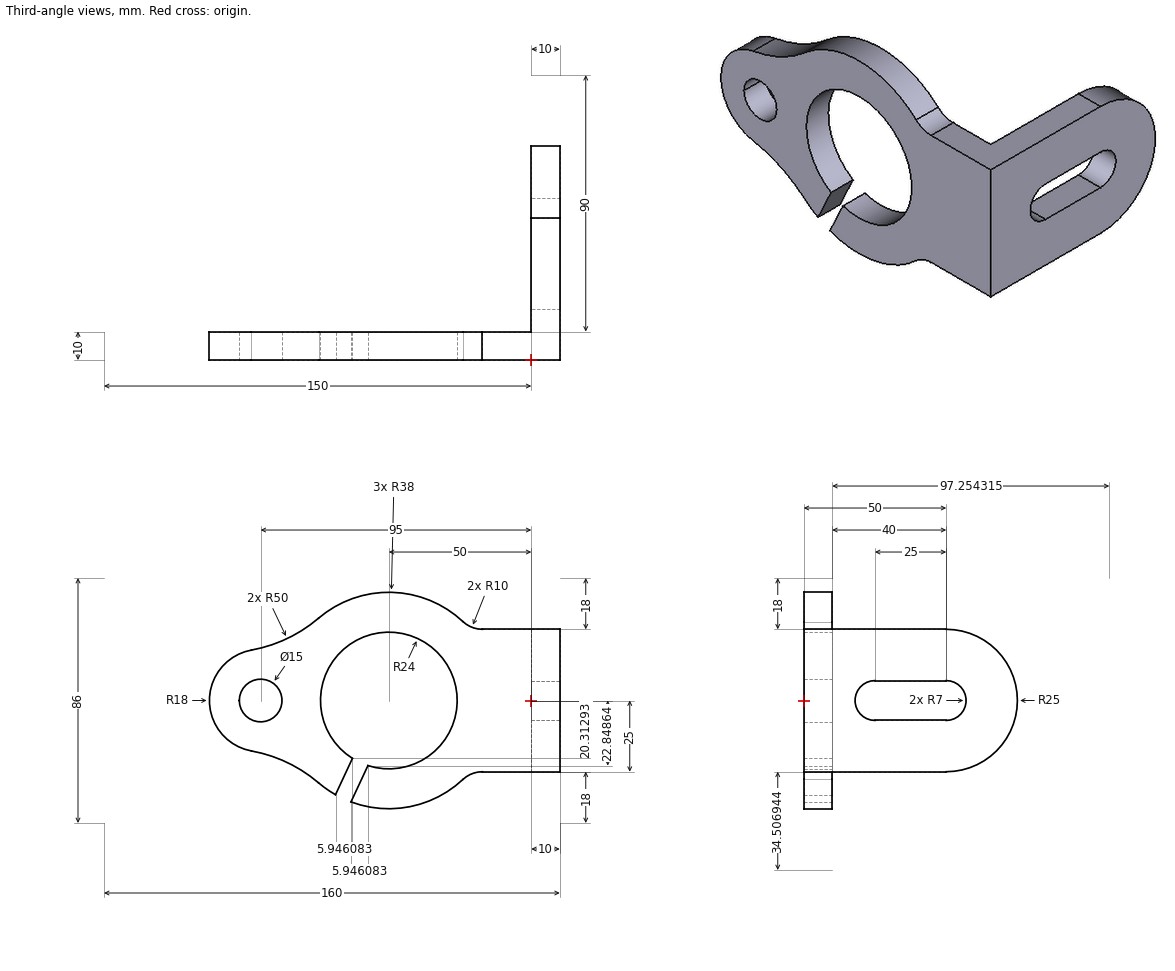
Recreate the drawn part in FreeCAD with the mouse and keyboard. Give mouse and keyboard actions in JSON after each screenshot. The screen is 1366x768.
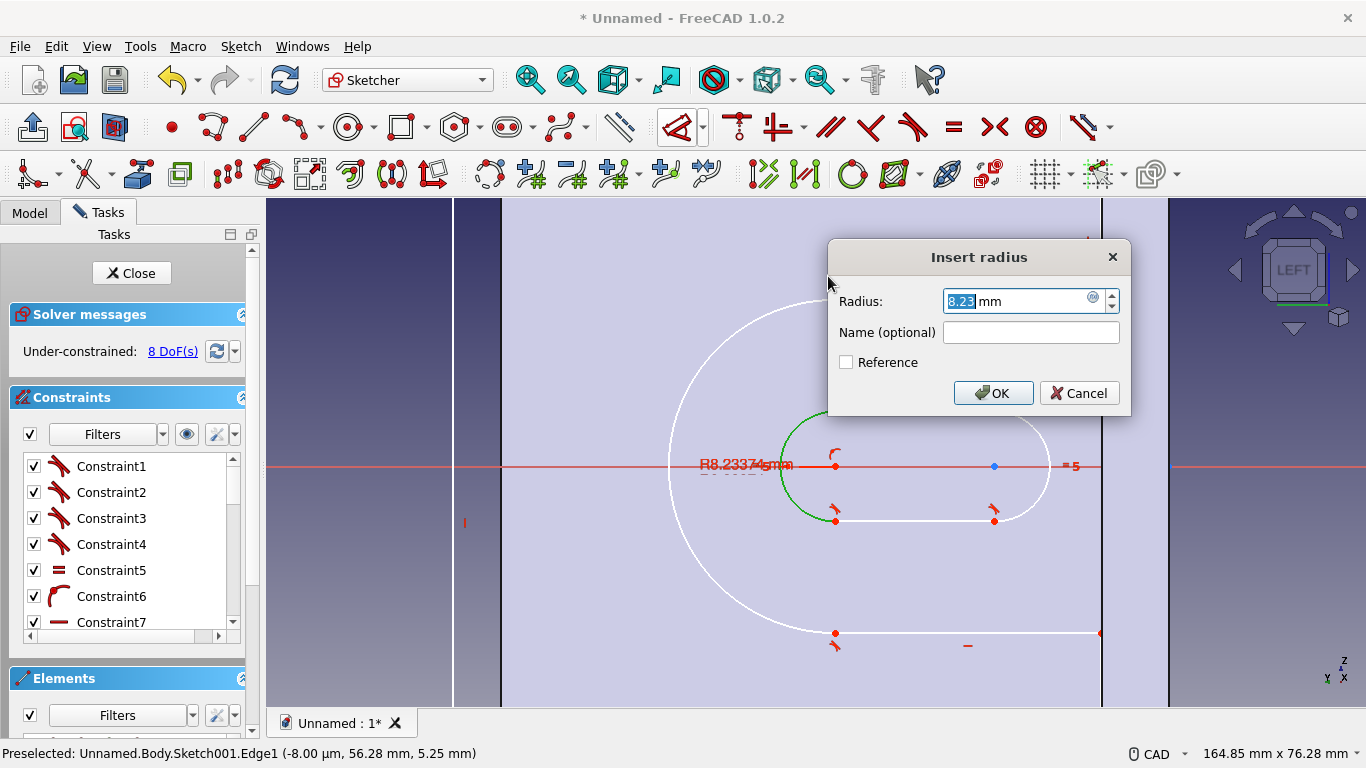
{"action": "type", "text": "7"}
{"action": "key", "text": "Return"}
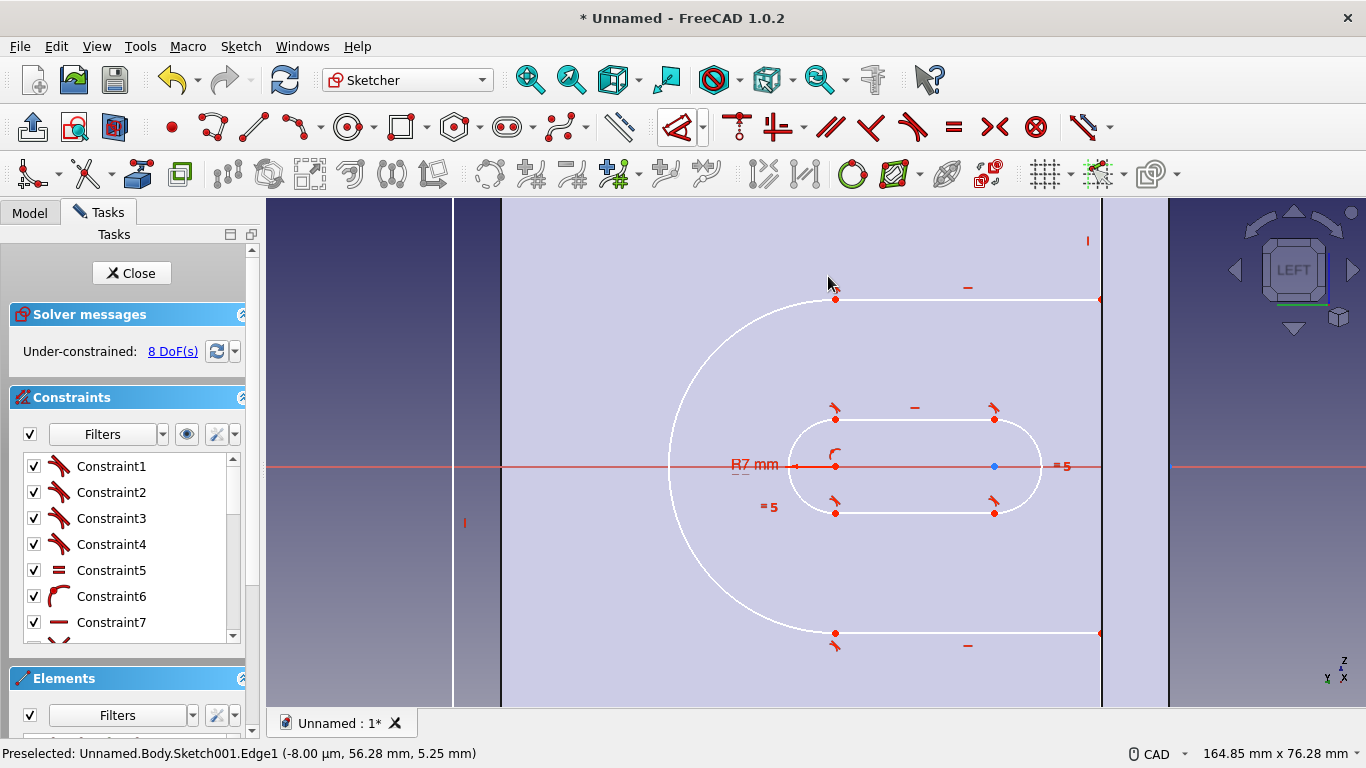
{"action": "left_click", "coordinate": [701, 369]}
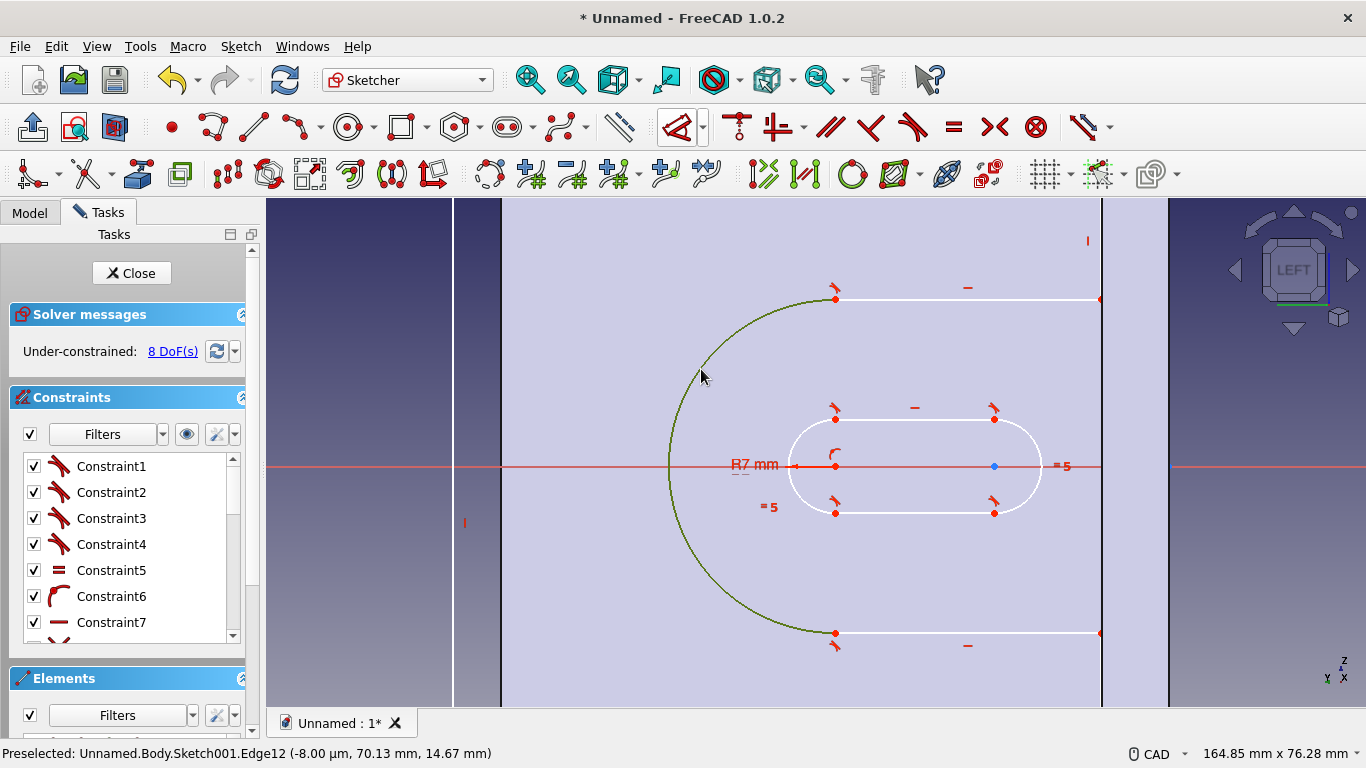
{"action": "left_click", "coordinate": [702, 128]}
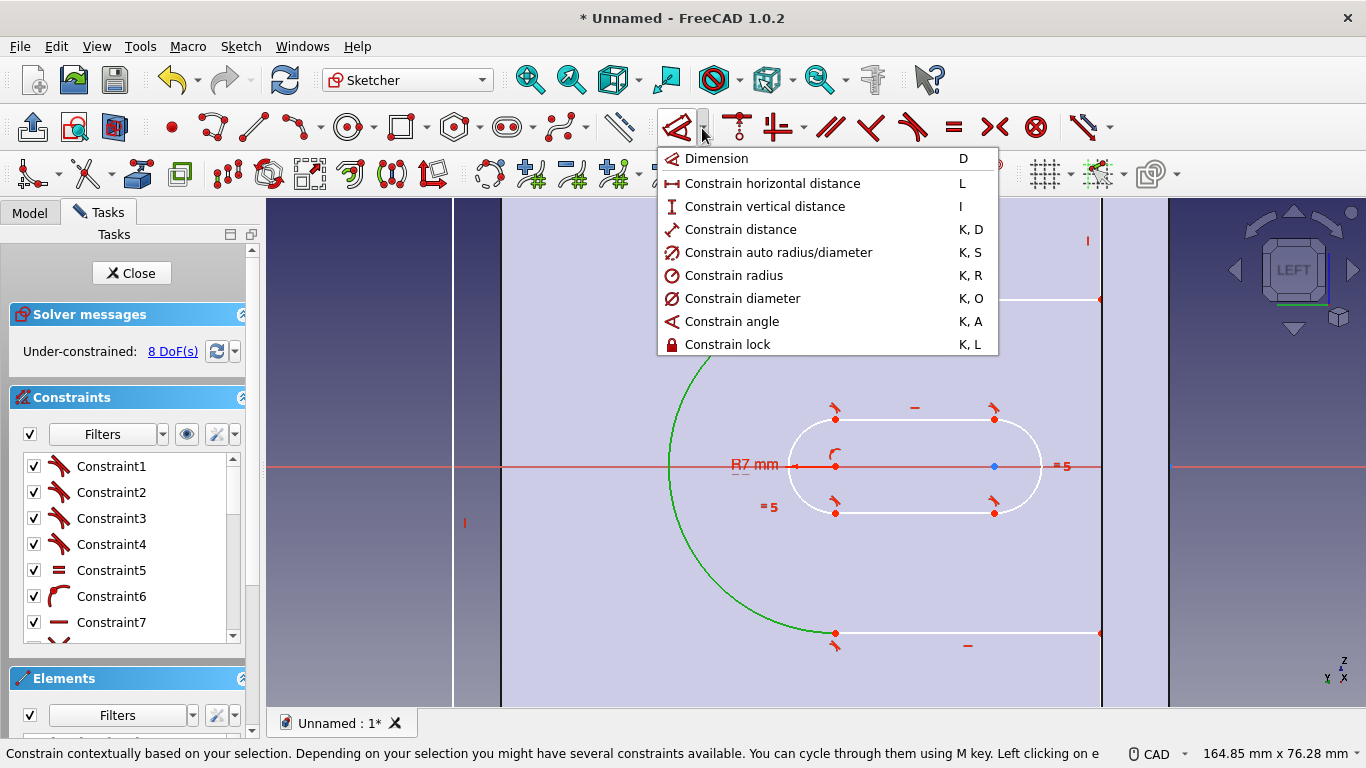
{"action": "left_click", "coordinate": [828, 276]}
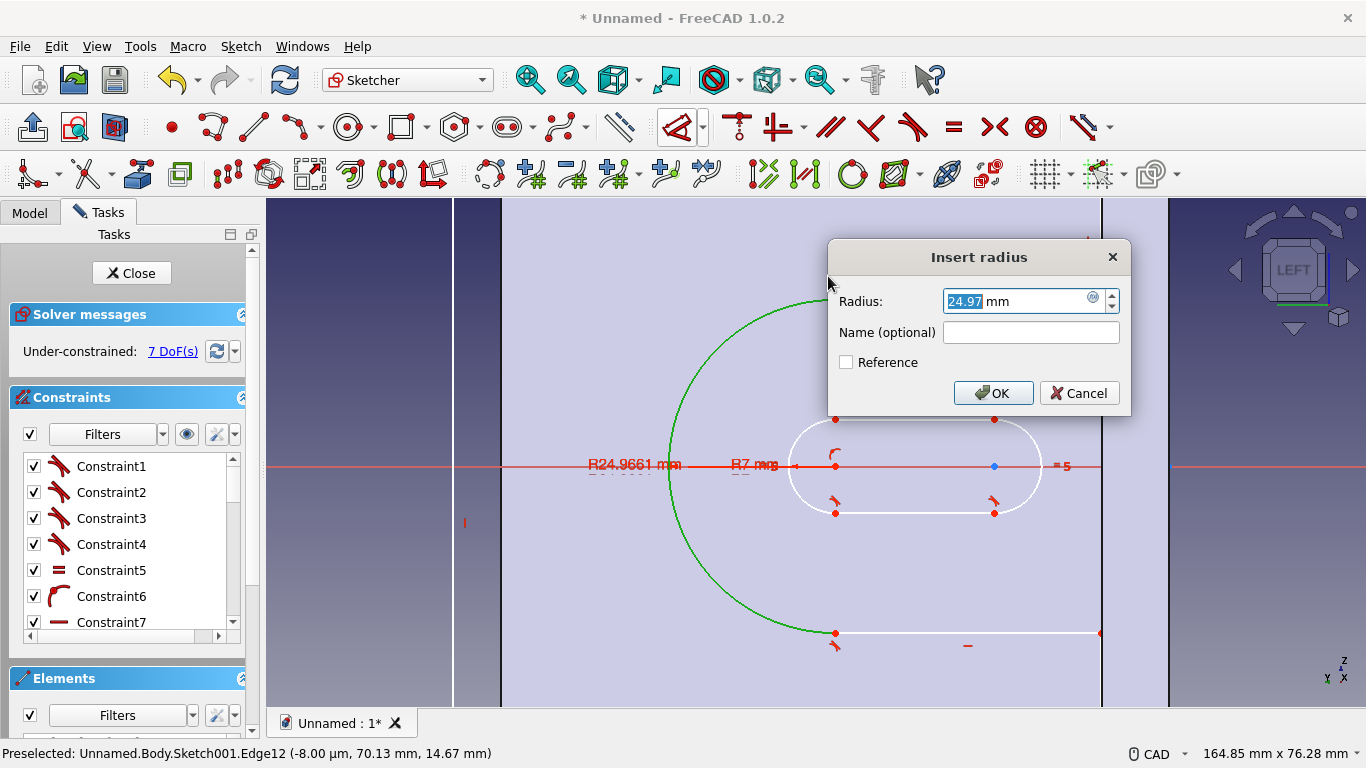
{"action": "type", "text": "25"}
{"action": "key", "text": "Return"}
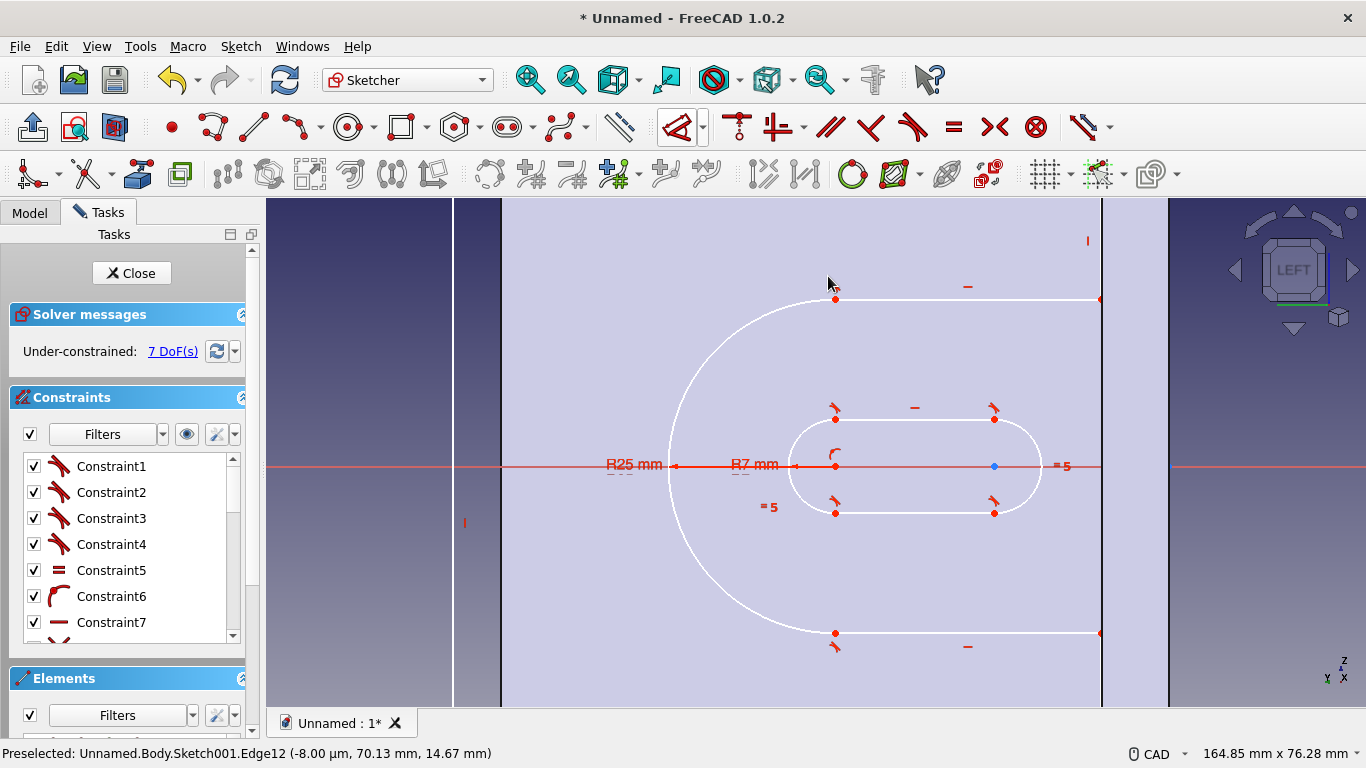
{"action": "left_click", "coordinate": [883, 420]}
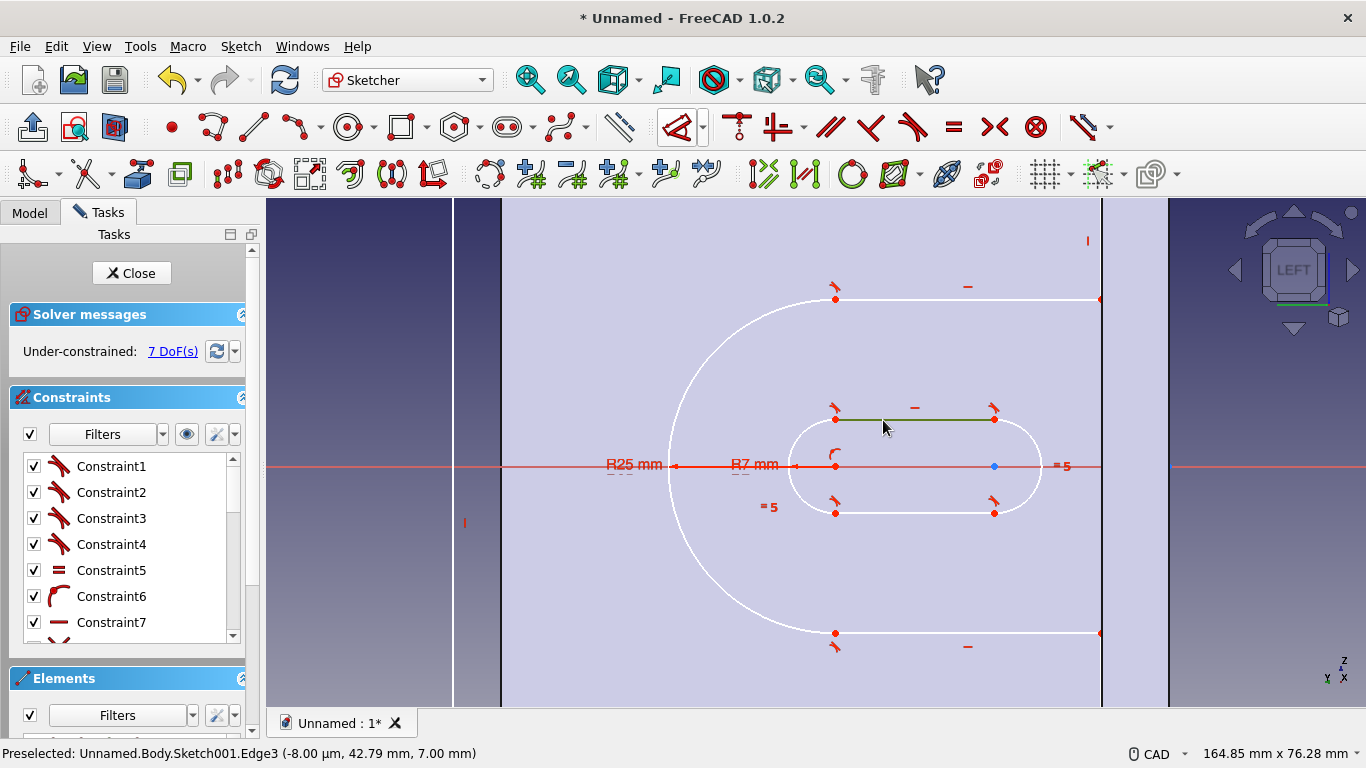
{"action": "key", "text": "l"}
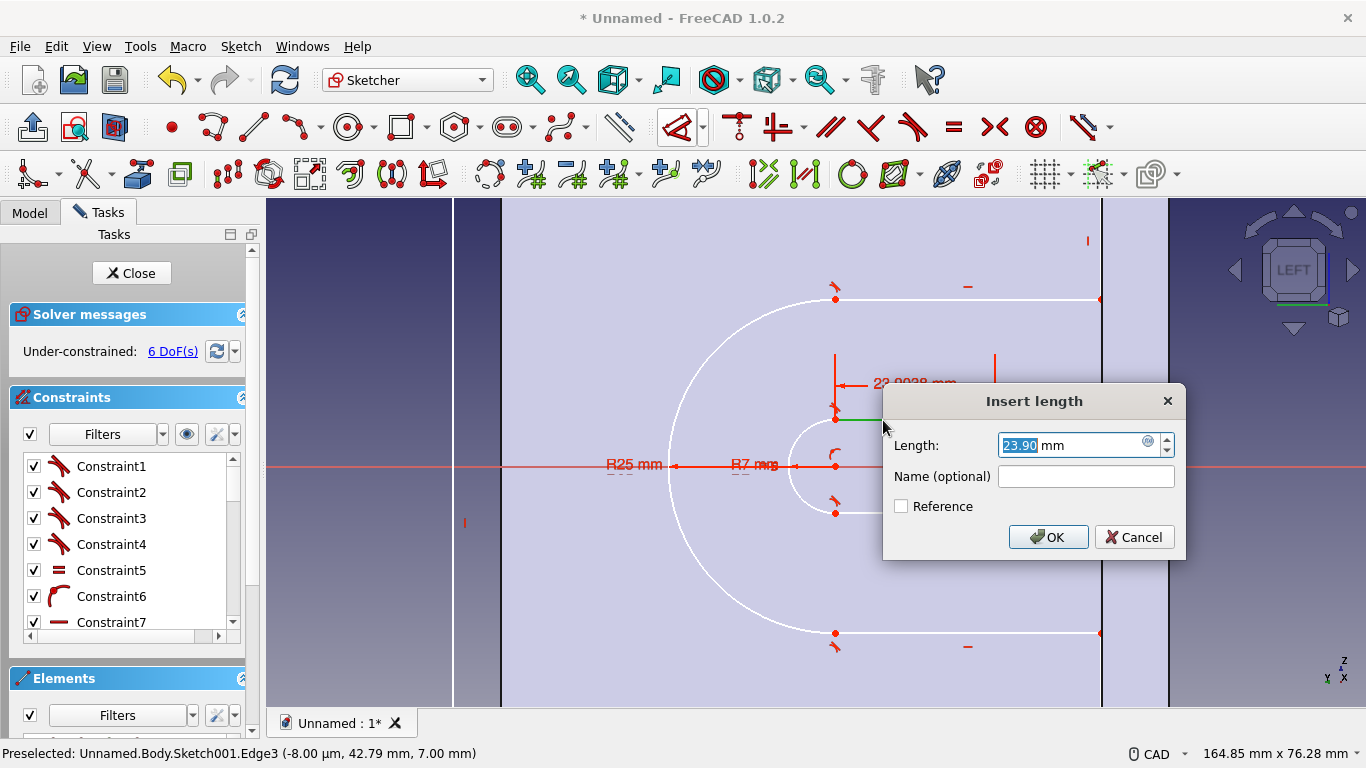
{"action": "type", "text": "25"}
{"action": "key", "text": "Return"}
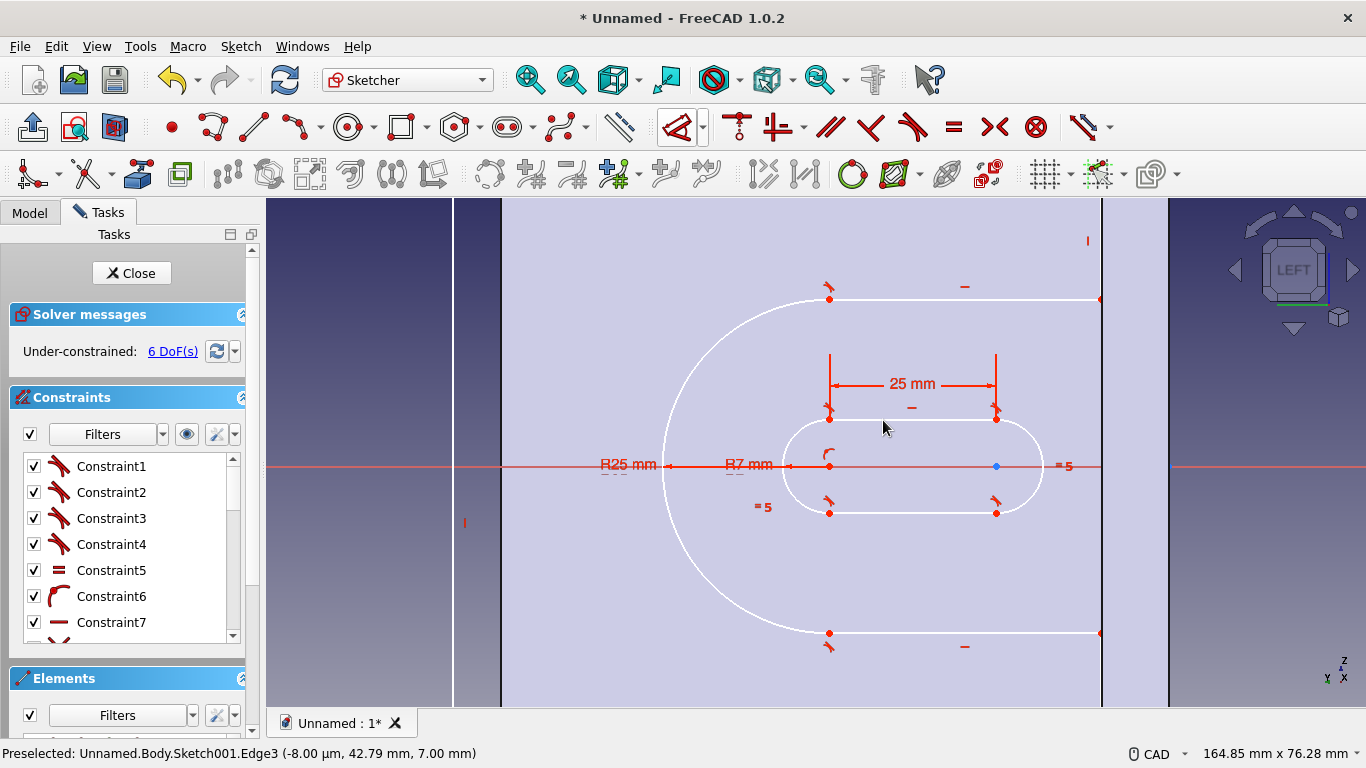
{"action": "left_click", "coordinate": [911, 300]}